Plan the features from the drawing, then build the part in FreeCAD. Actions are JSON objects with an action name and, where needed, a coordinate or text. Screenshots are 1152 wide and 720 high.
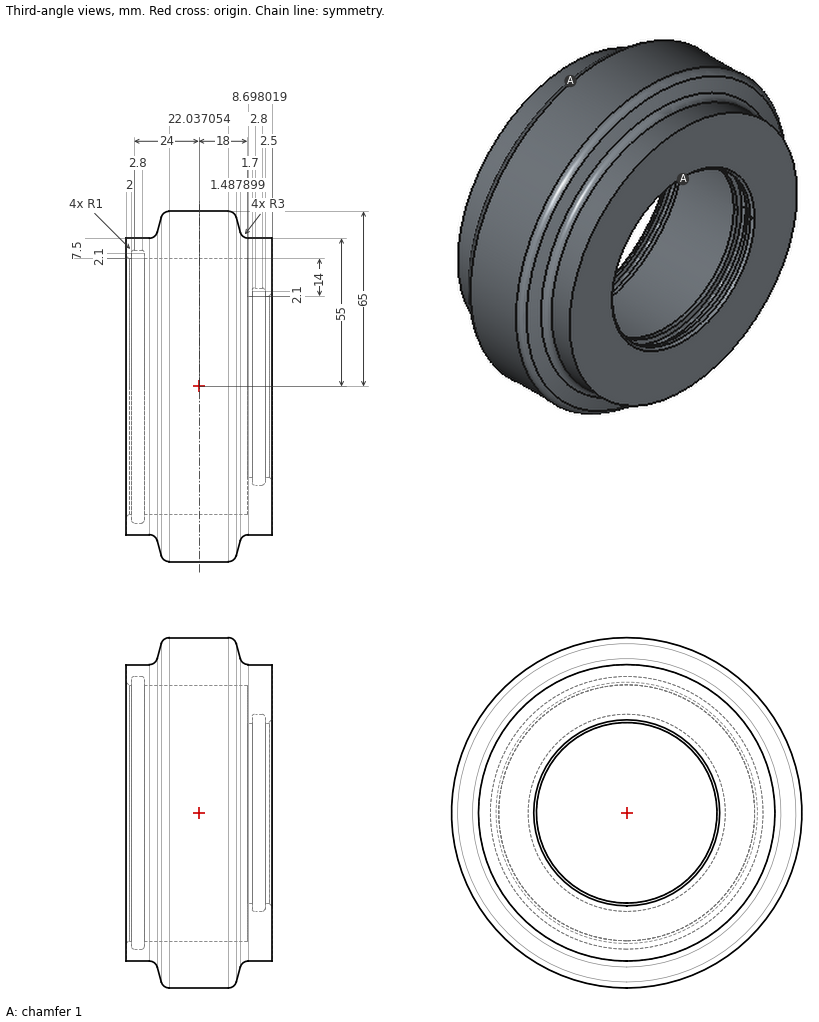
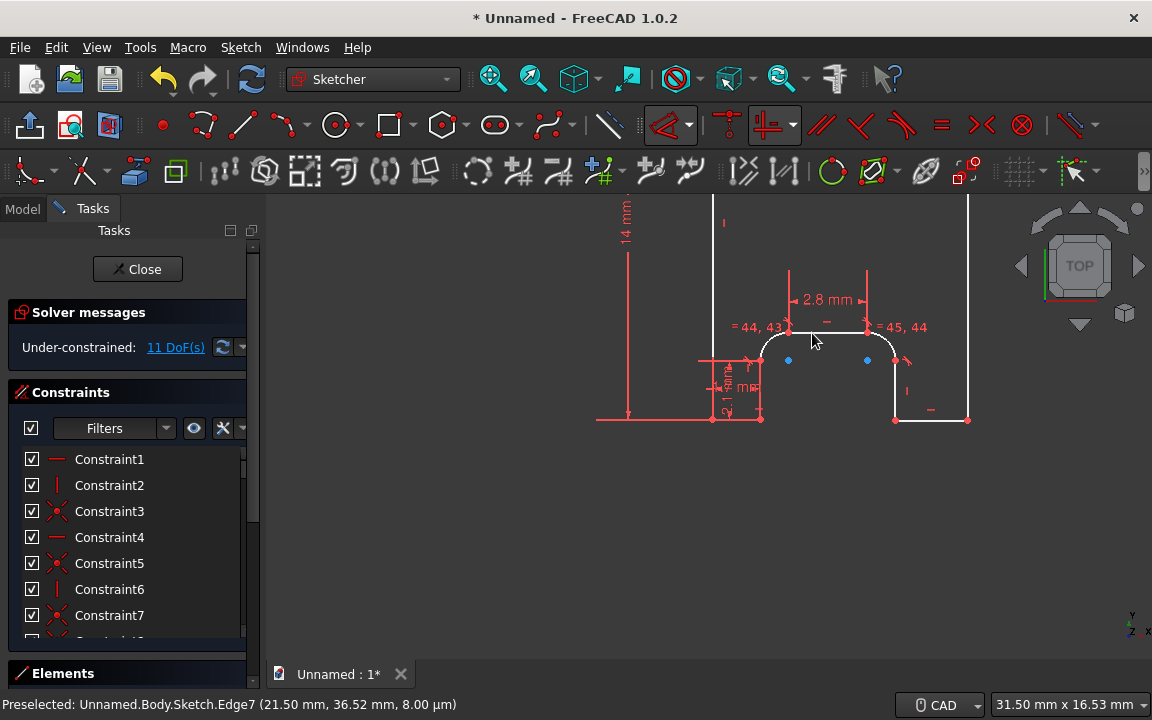
{"action": "left_click", "coordinate": [895, 379]}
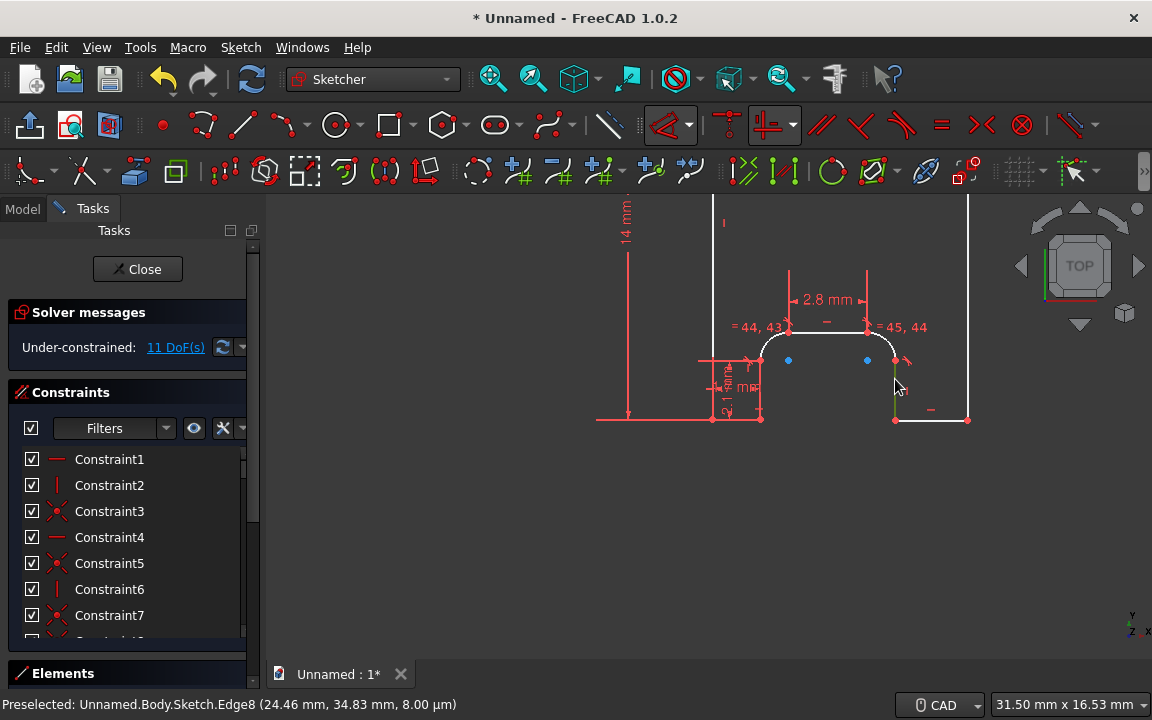
{"action": "key", "text": "i"}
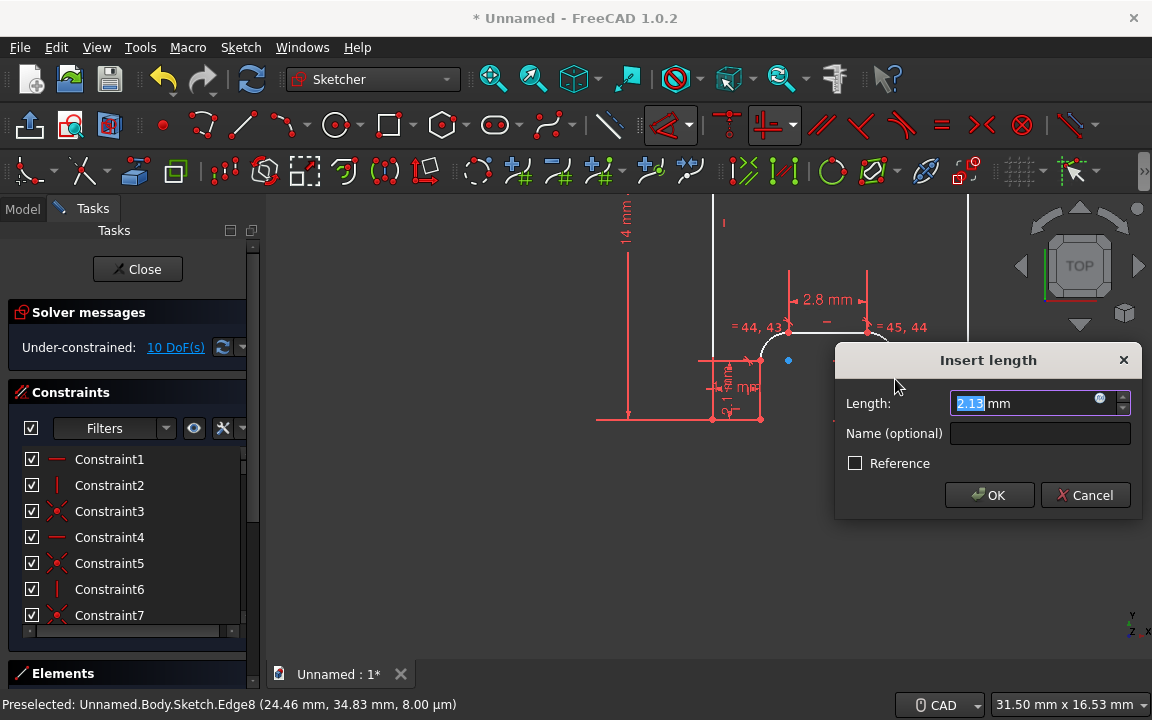
{"action": "type", "text": "2.1"}
{"action": "key", "text": "Return"}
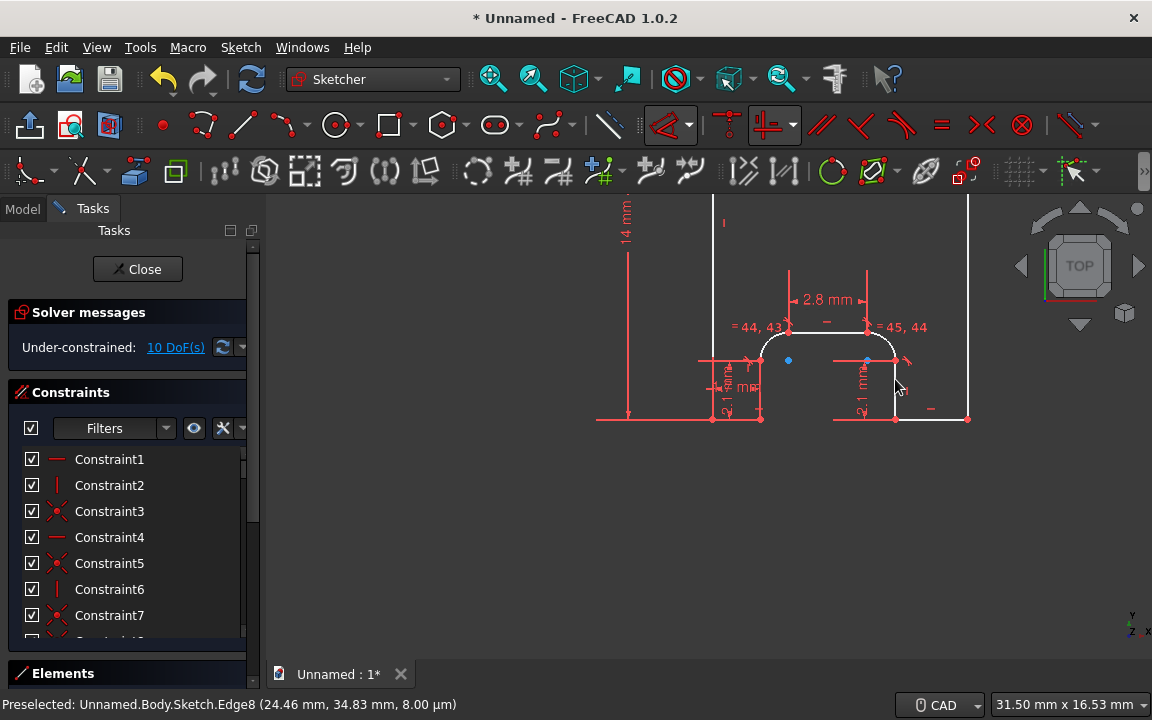
{"action": "left_click", "coordinate": [917, 420]}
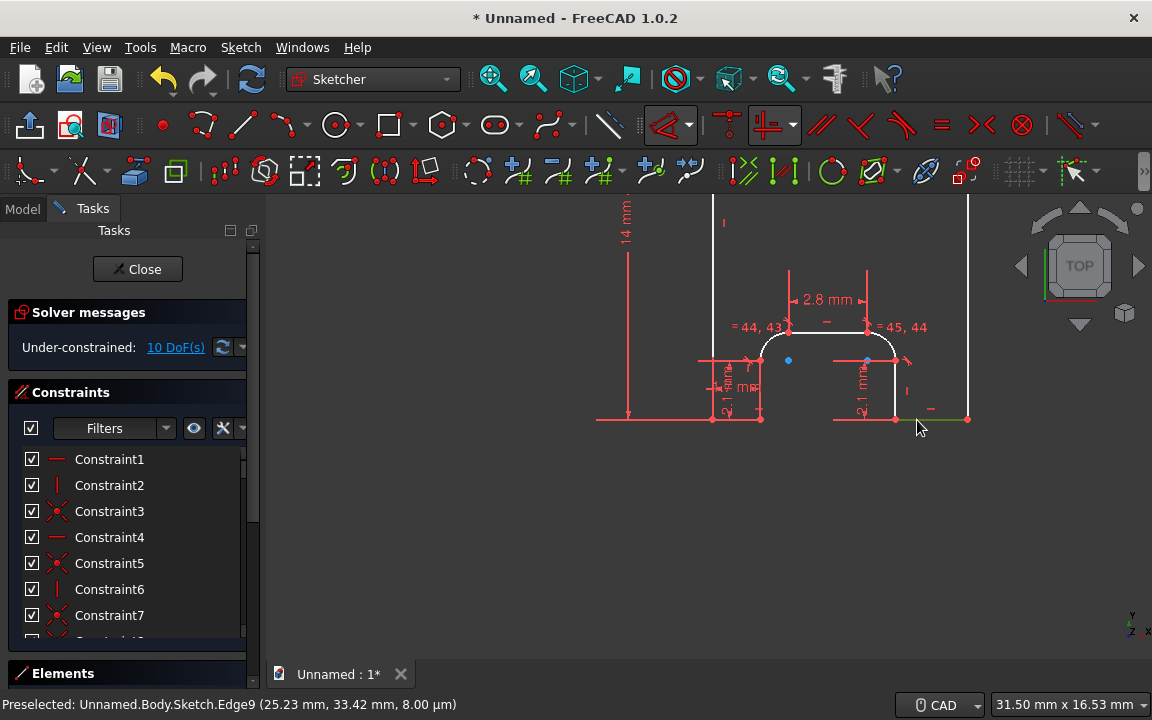
{"action": "key", "text": "l"}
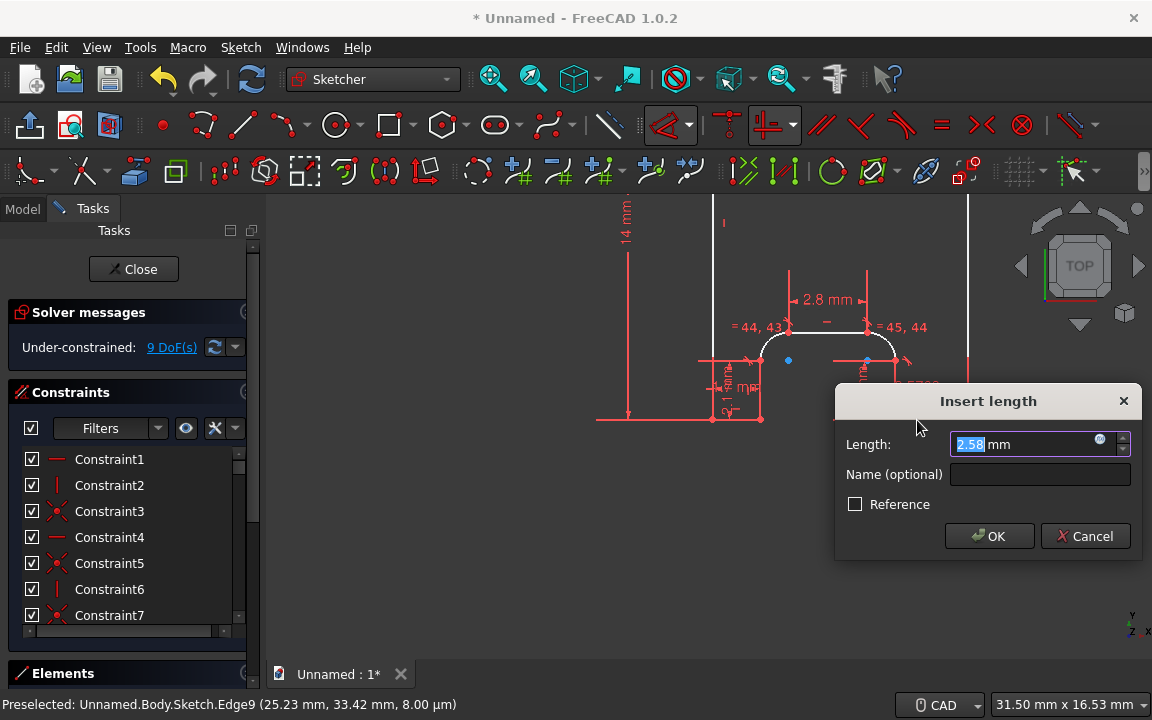
{"action": "type", "text": "2.5"}
{"action": "key", "text": "Return"}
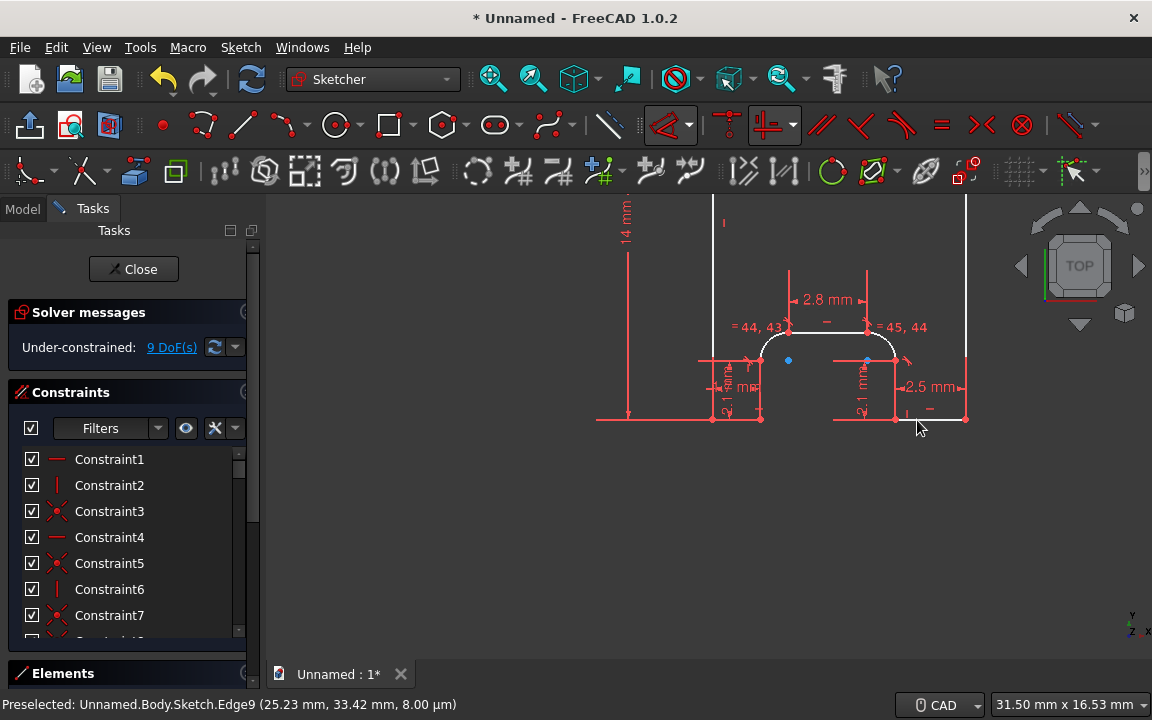
{"action": "scroll", "coordinate": [726, 423], "scroll_direction": "down", "scroll_amount": 9}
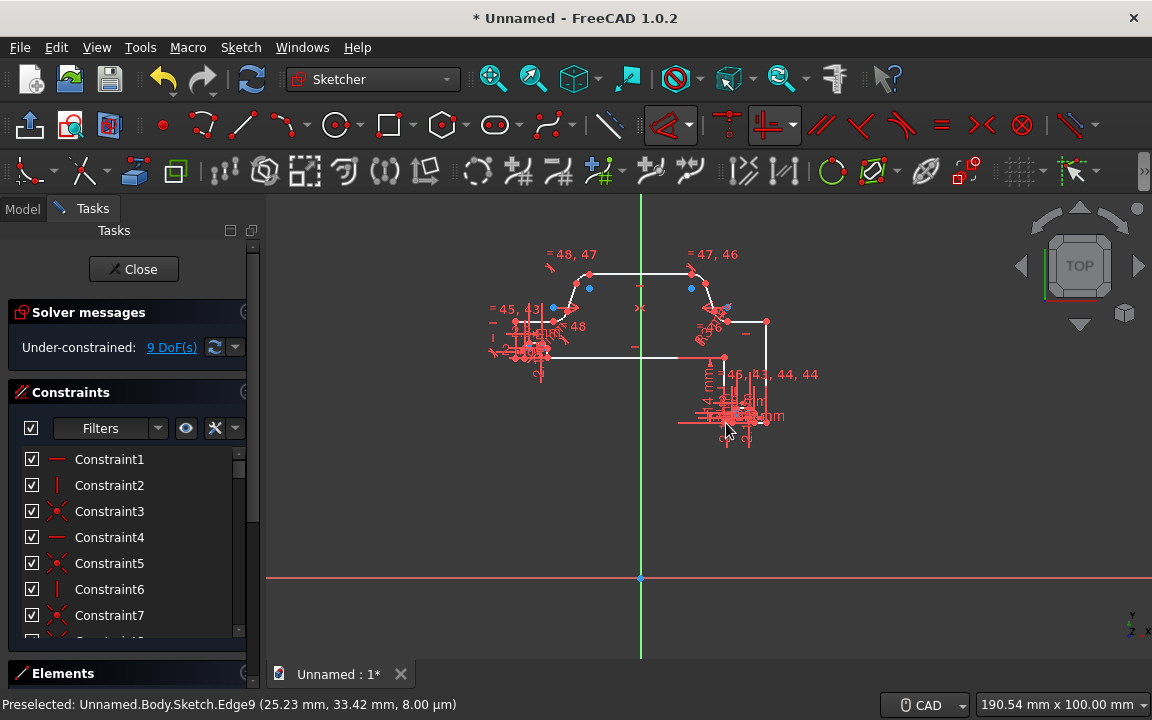
{"action": "scroll", "coordinate": [516, 333], "scroll_direction": "up", "scroll_amount": 2}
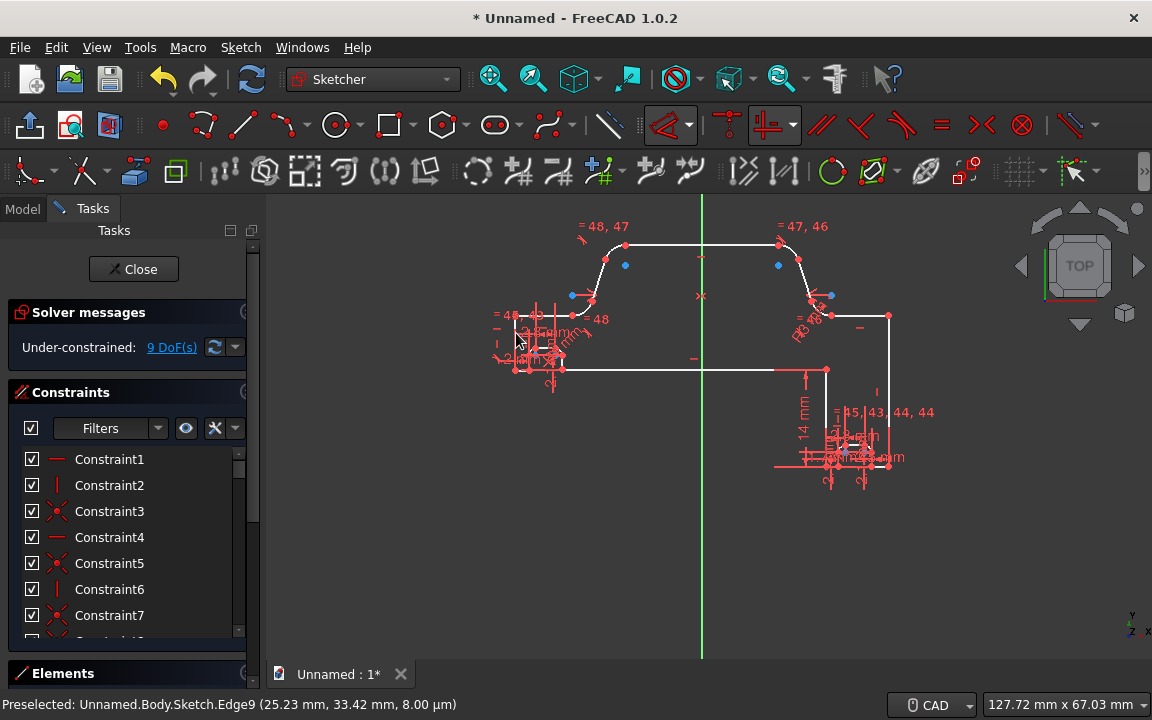
{"action": "scroll", "coordinate": [515, 332], "scroll_direction": "up", "scroll_amount": 4}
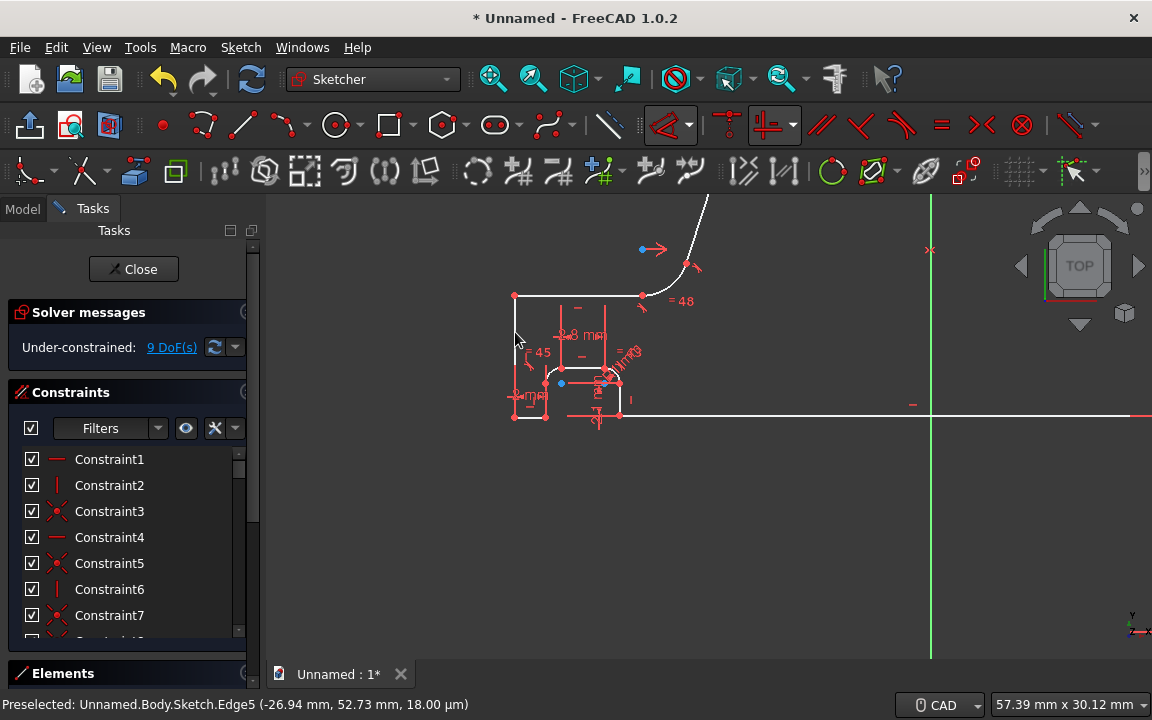
{"action": "left_click", "coordinate": [515, 332]}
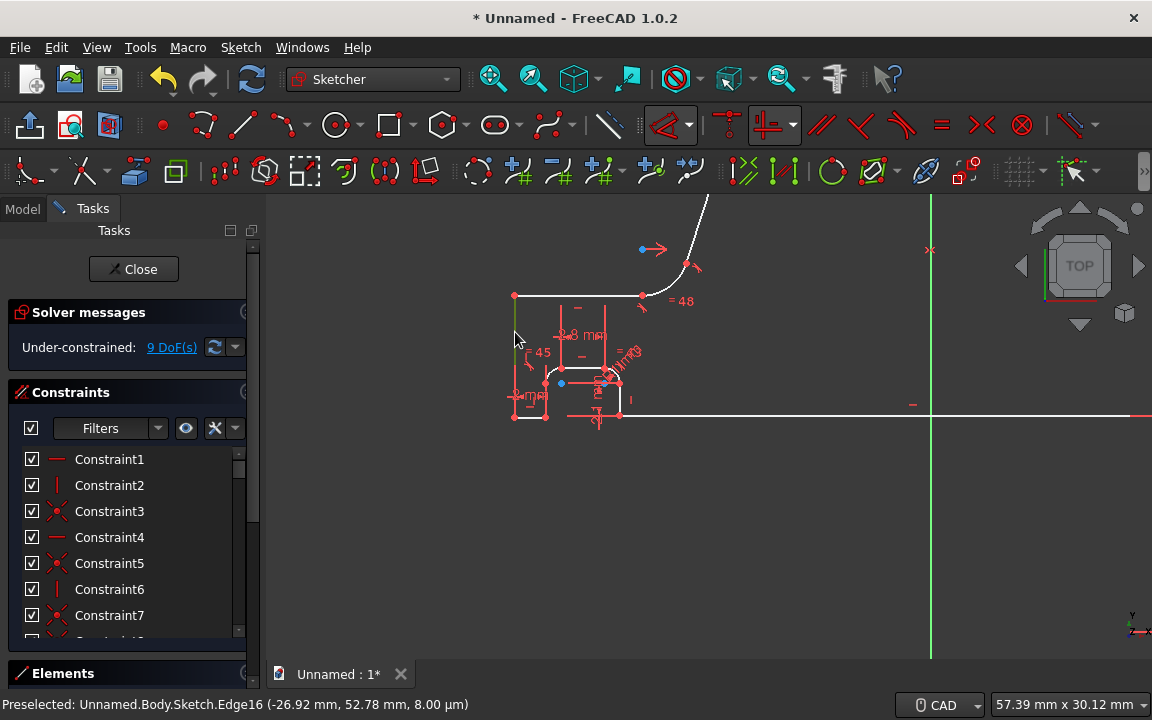
{"action": "key", "text": "i"}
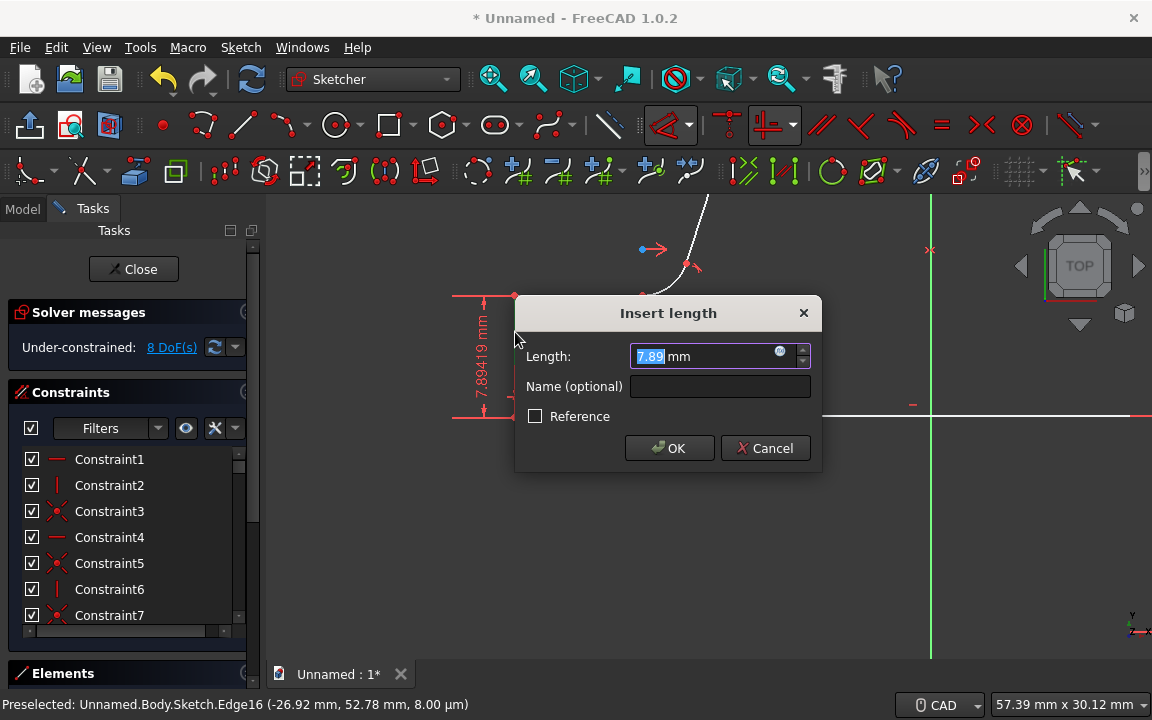
{"action": "type", "text": "7.5"}
{"action": "key", "text": "Return"}